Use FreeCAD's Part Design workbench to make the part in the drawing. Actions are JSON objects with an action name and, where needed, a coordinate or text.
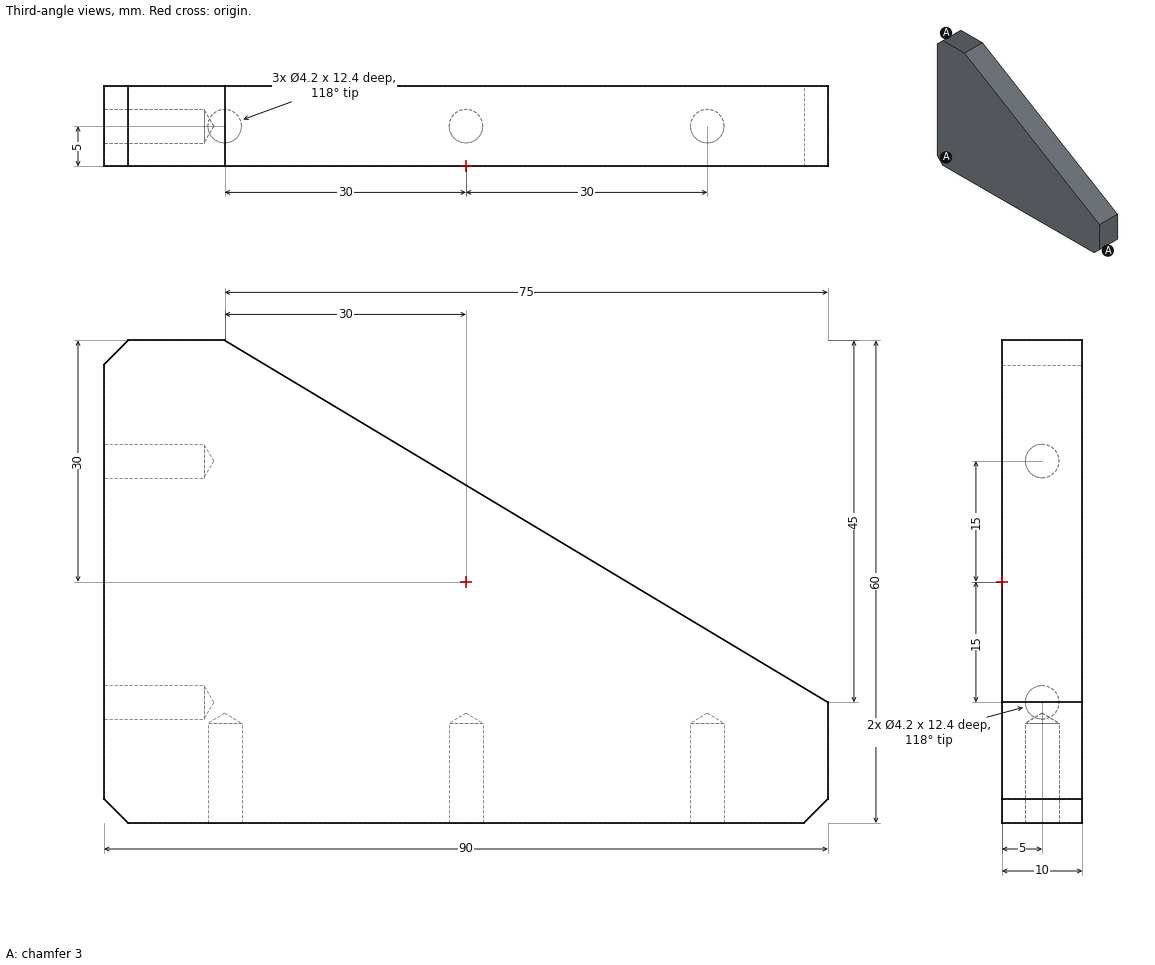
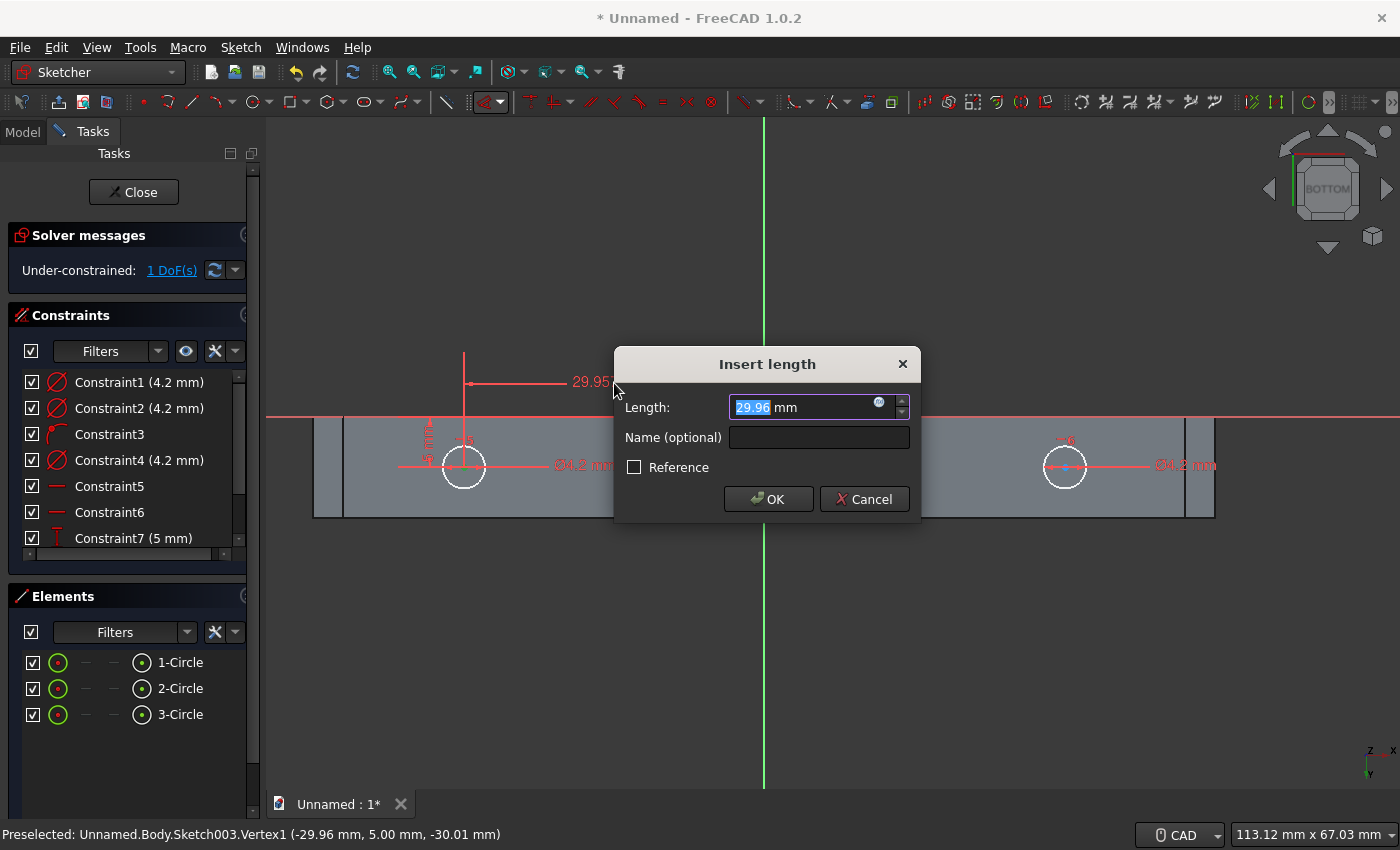
{"action": "type", "text": "30"}
{"action": "key", "text": "Return"}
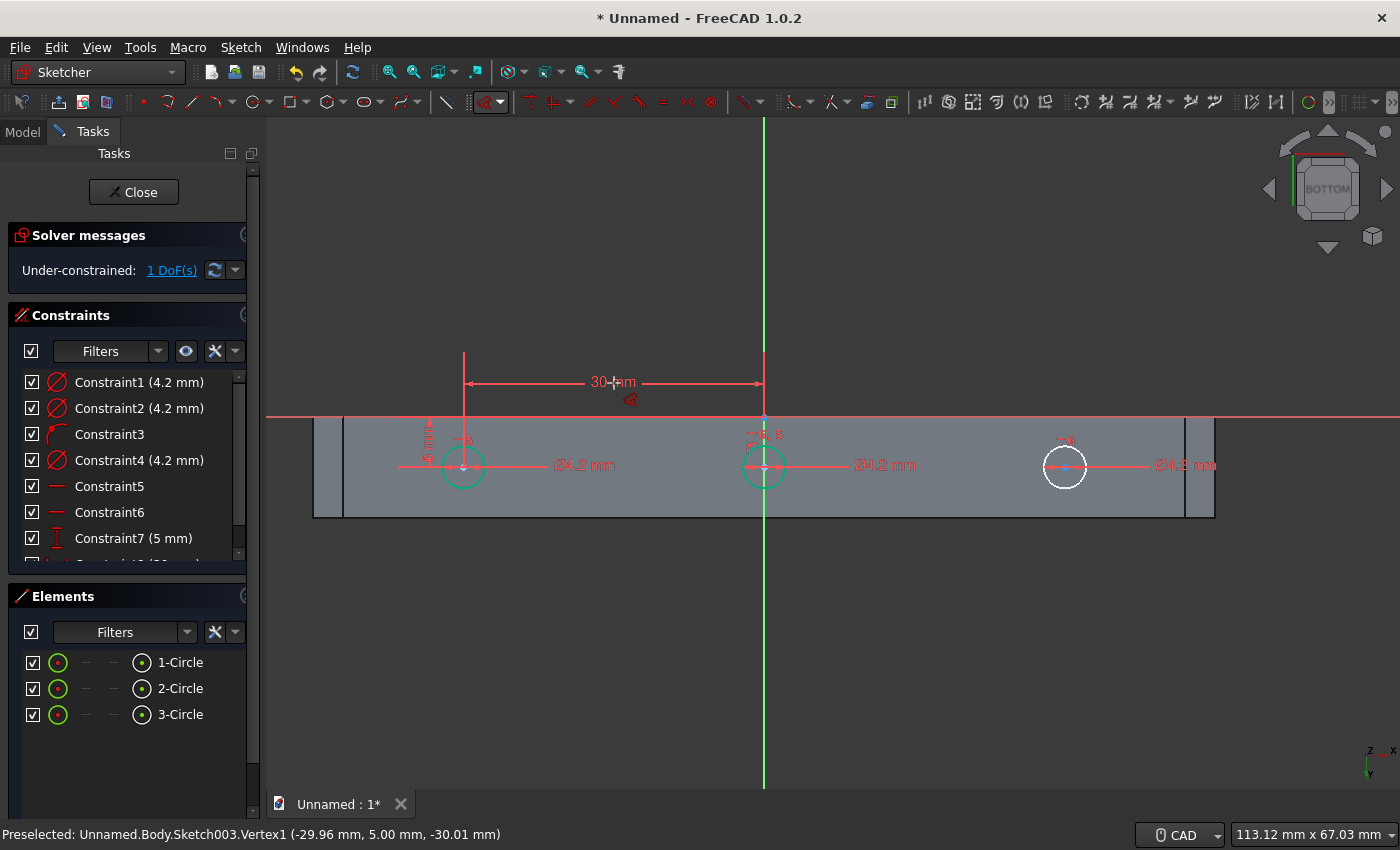
{"action": "left_click", "coordinate": [1065, 467]}
{"action": "left_click", "coordinate": [915, 383]}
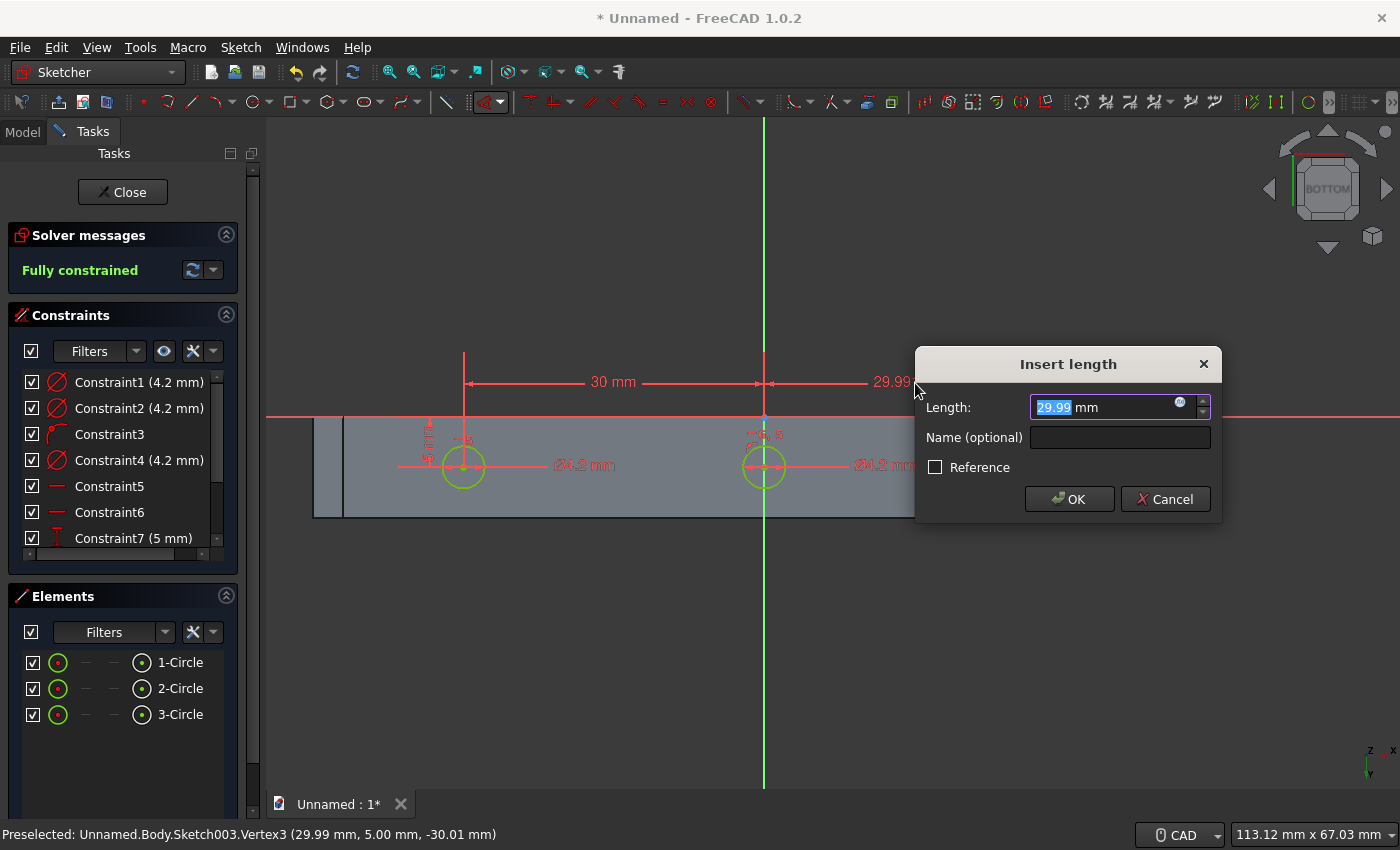
{"action": "type", "text": "30"}
{"action": "key", "text": "Return"}
{"action": "key", "text": "Escape"}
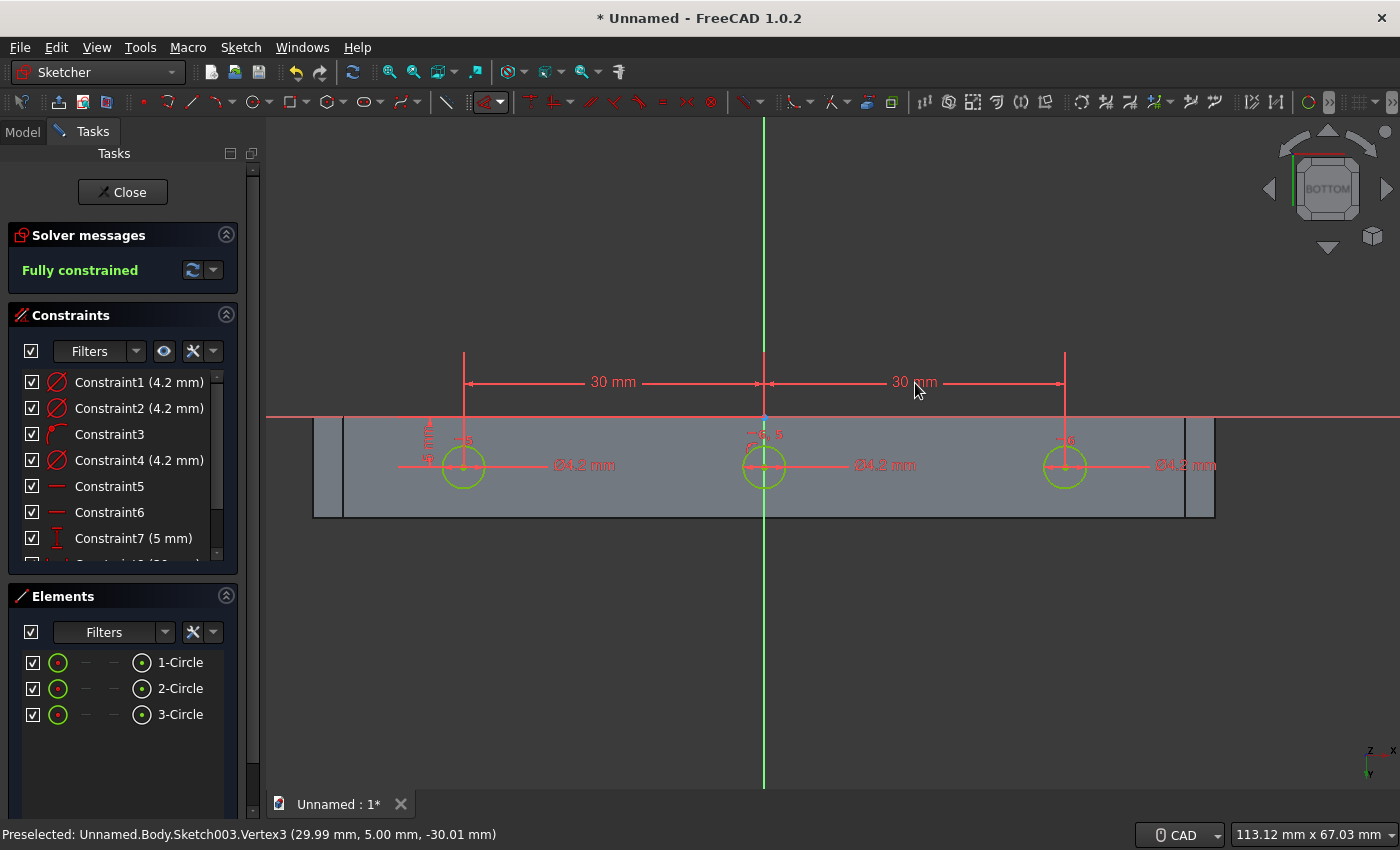
{"action": "left_click", "coordinate": [123, 192]}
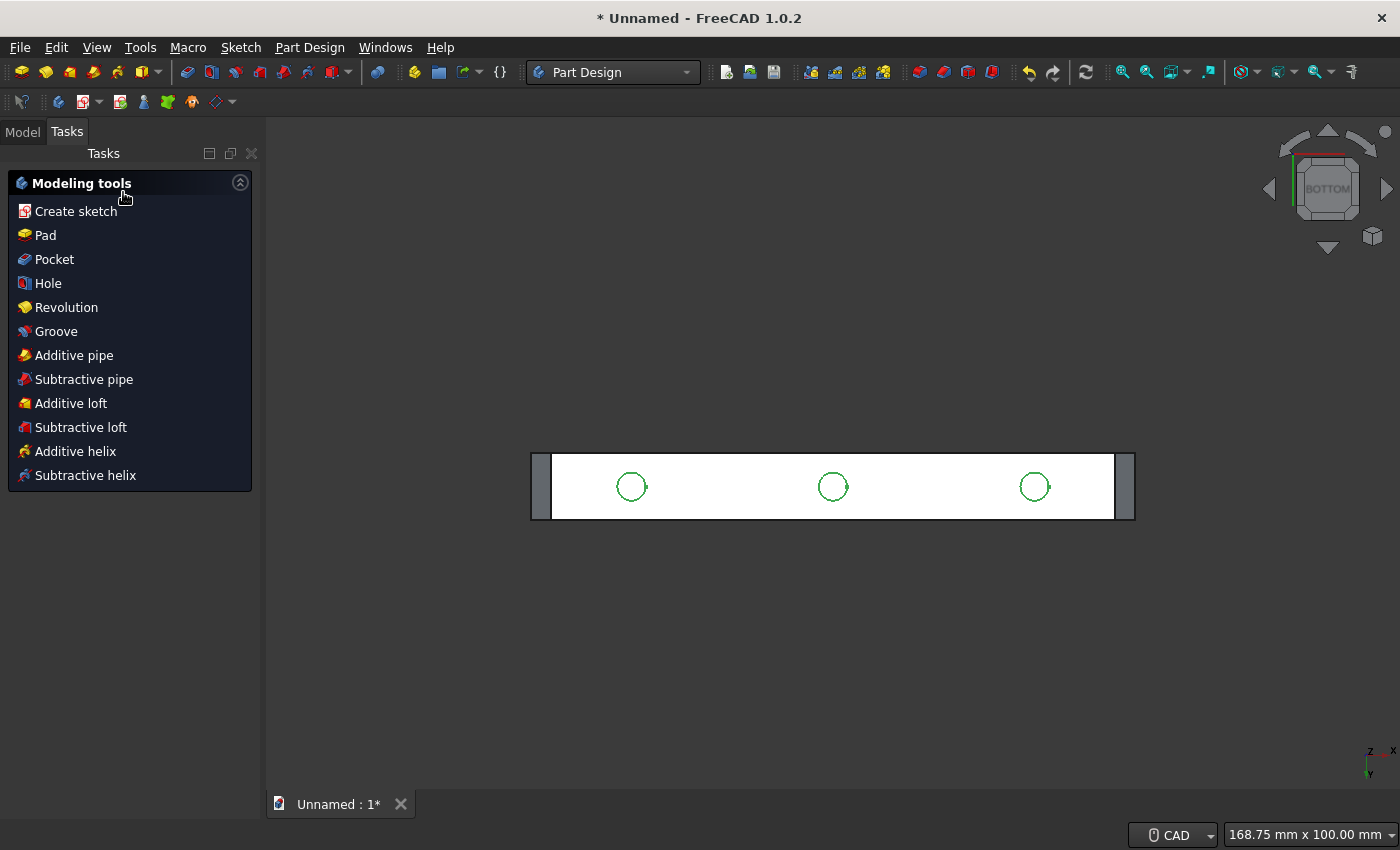
{"action": "left_click", "coordinate": [212, 72]}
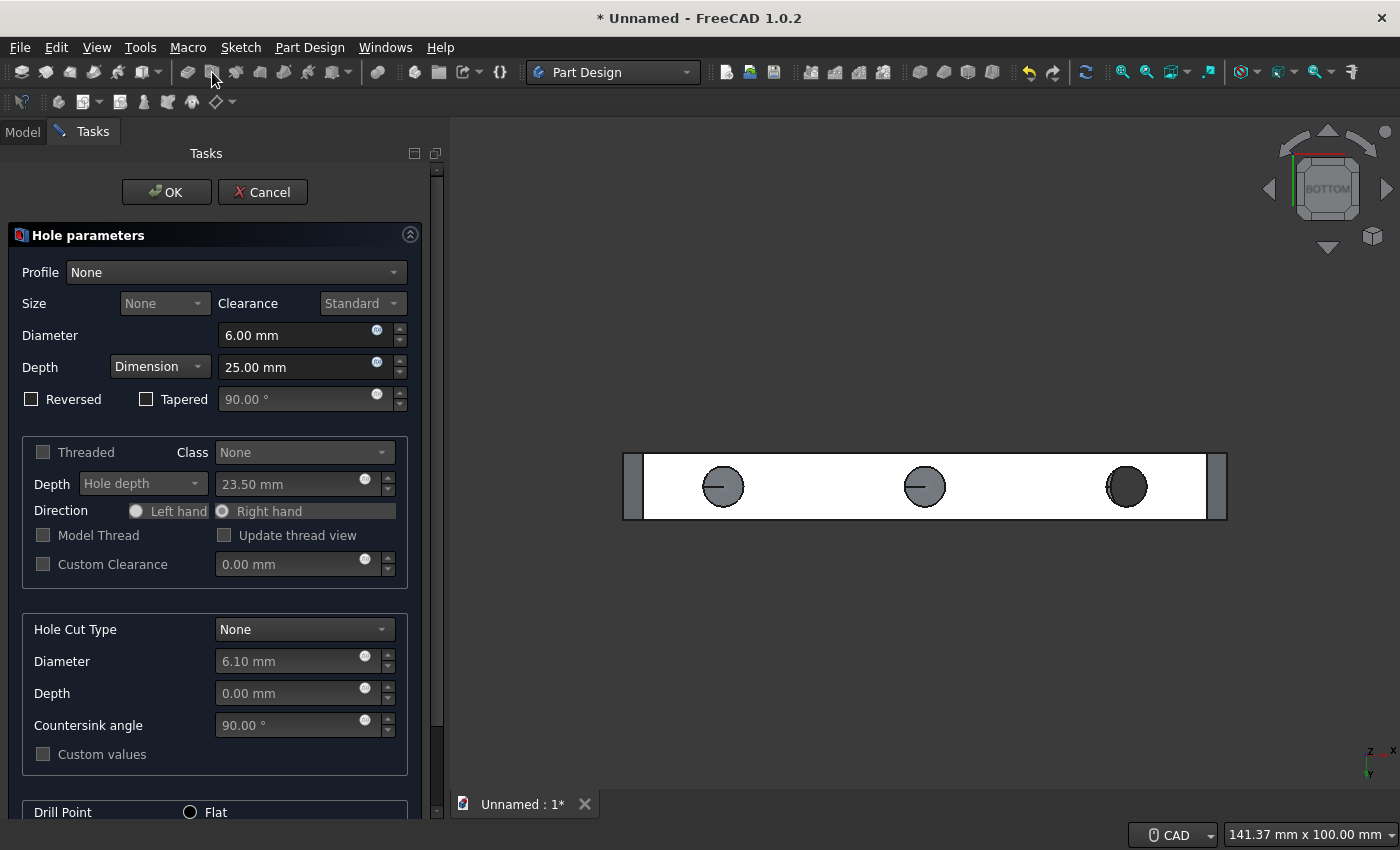
{"action": "triple_click", "coordinate": [305, 335]}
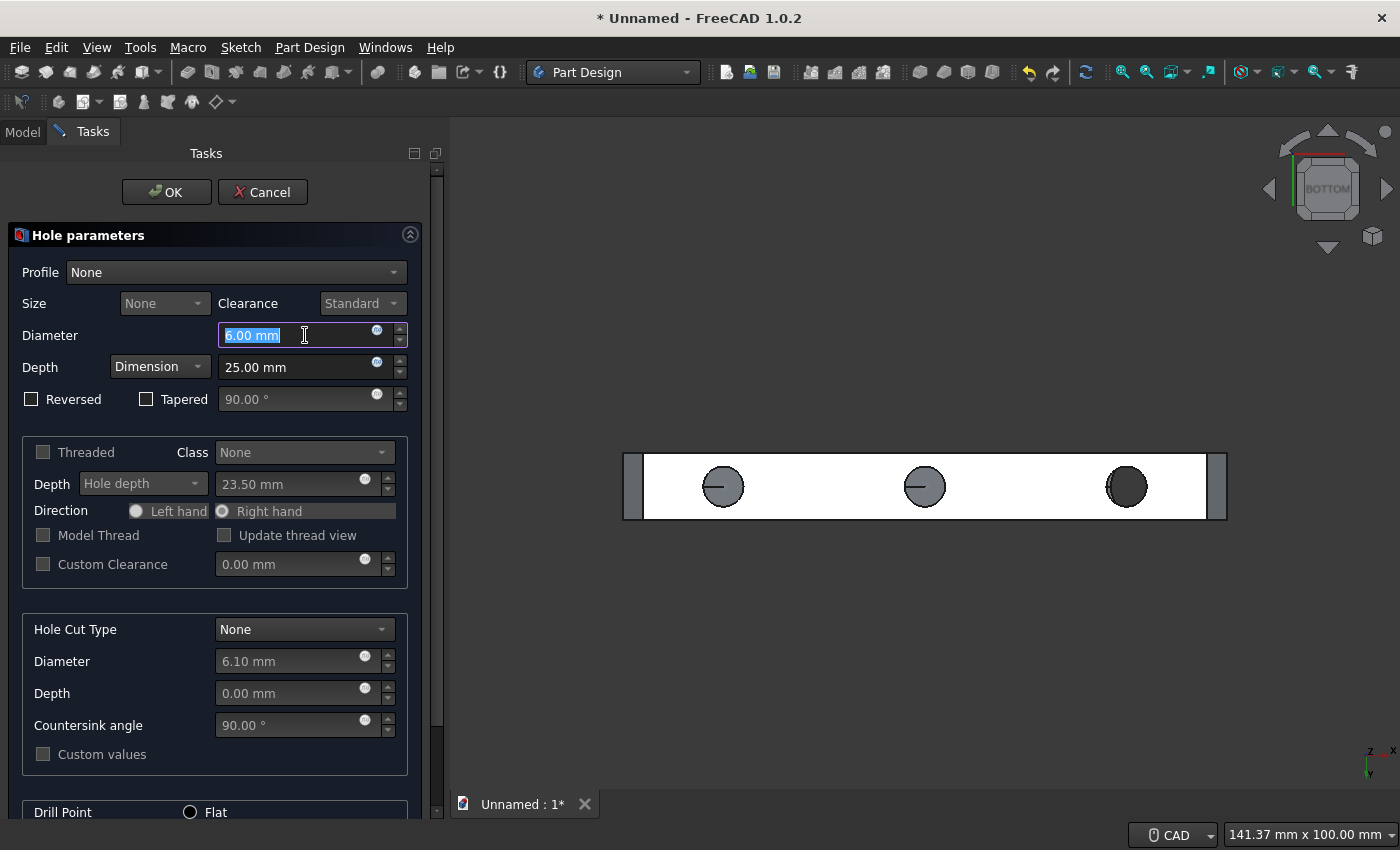
{"action": "type", "text": "4.2"}
{"action": "key", "text": "Tab"}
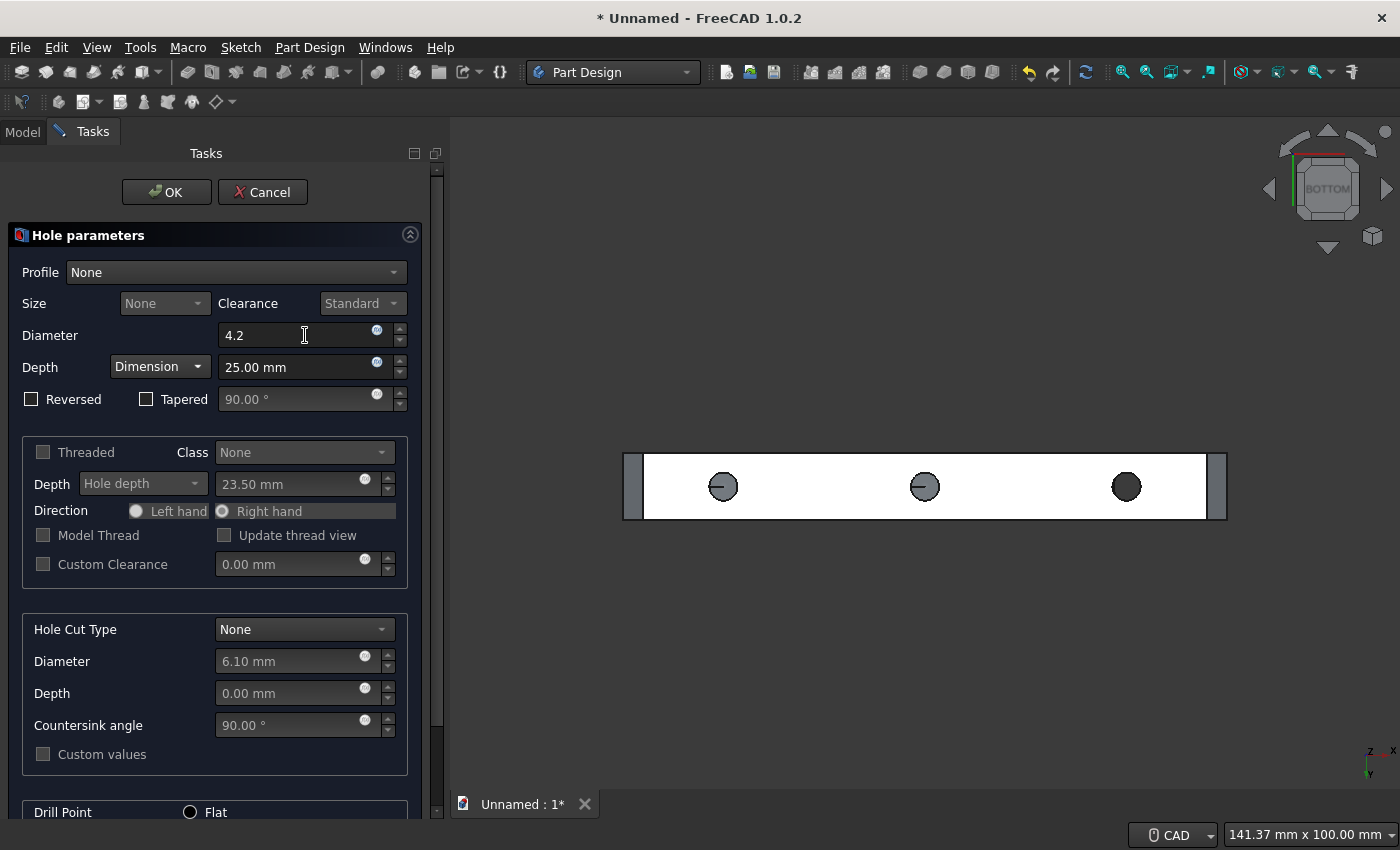
{"action": "triple_click", "coordinate": [305, 367]}